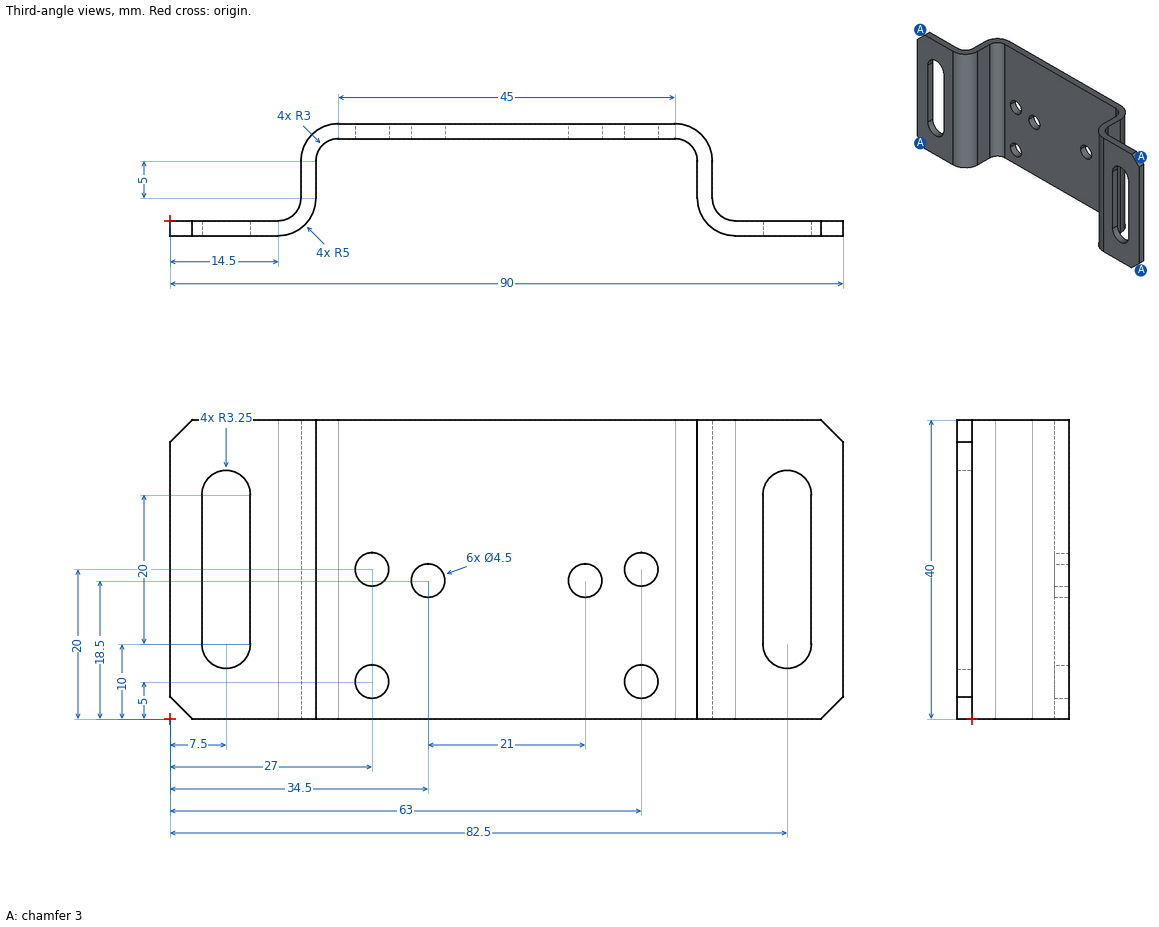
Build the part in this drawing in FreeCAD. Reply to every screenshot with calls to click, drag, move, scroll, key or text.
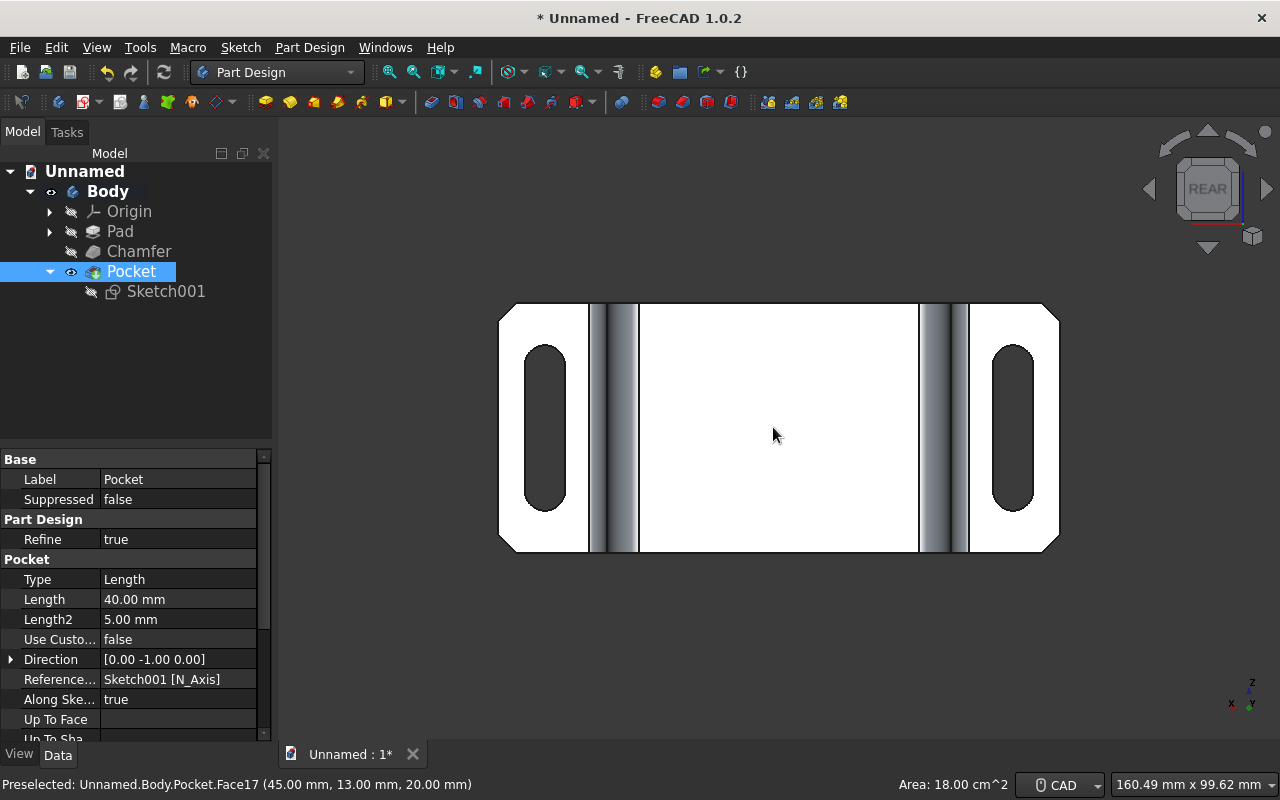
click(84, 102)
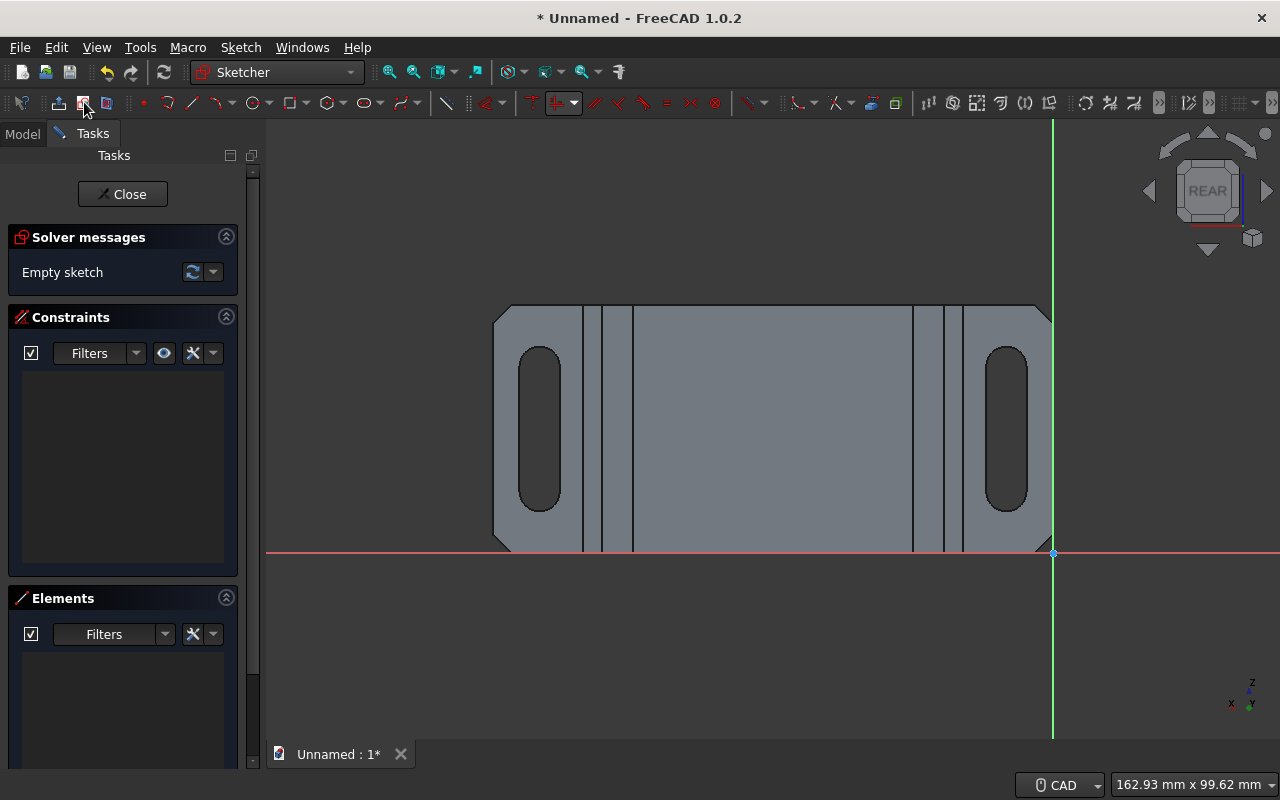
scroll(1115, 597, up, 2)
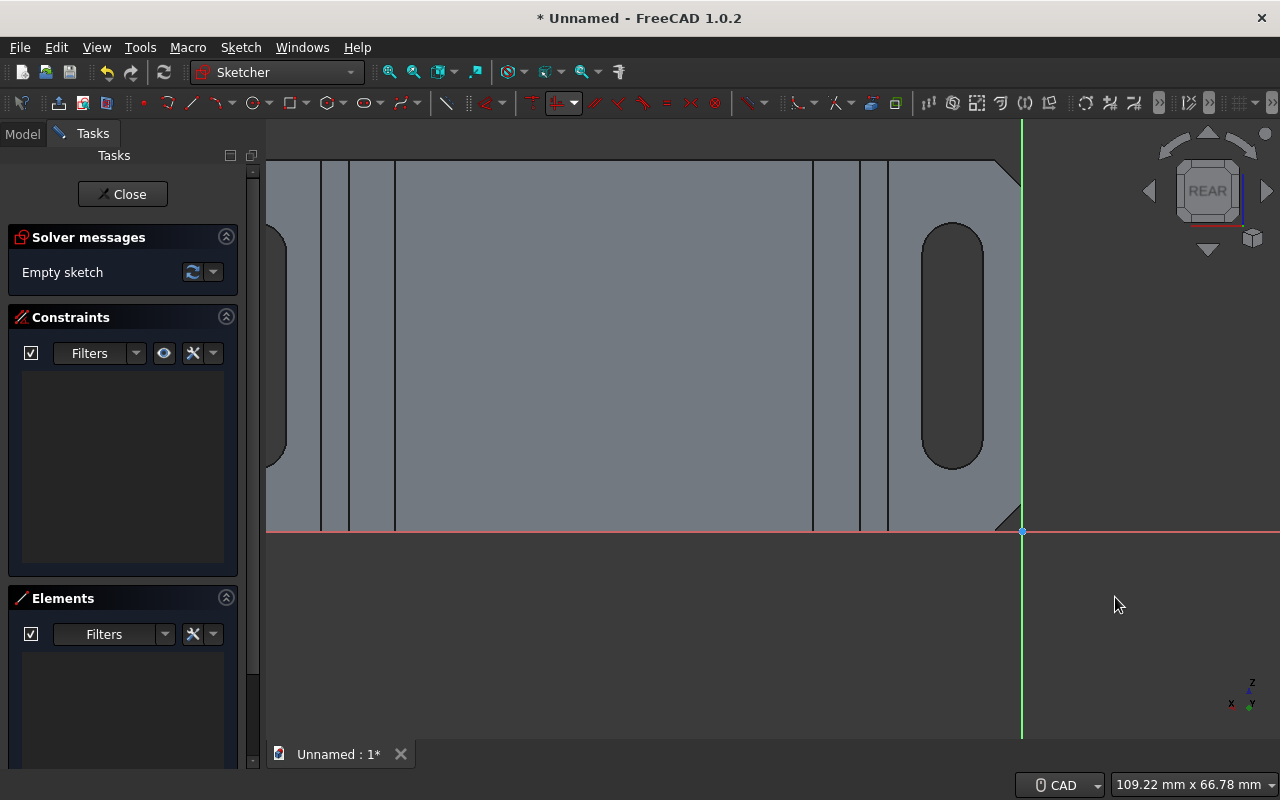
key(g)
key(c)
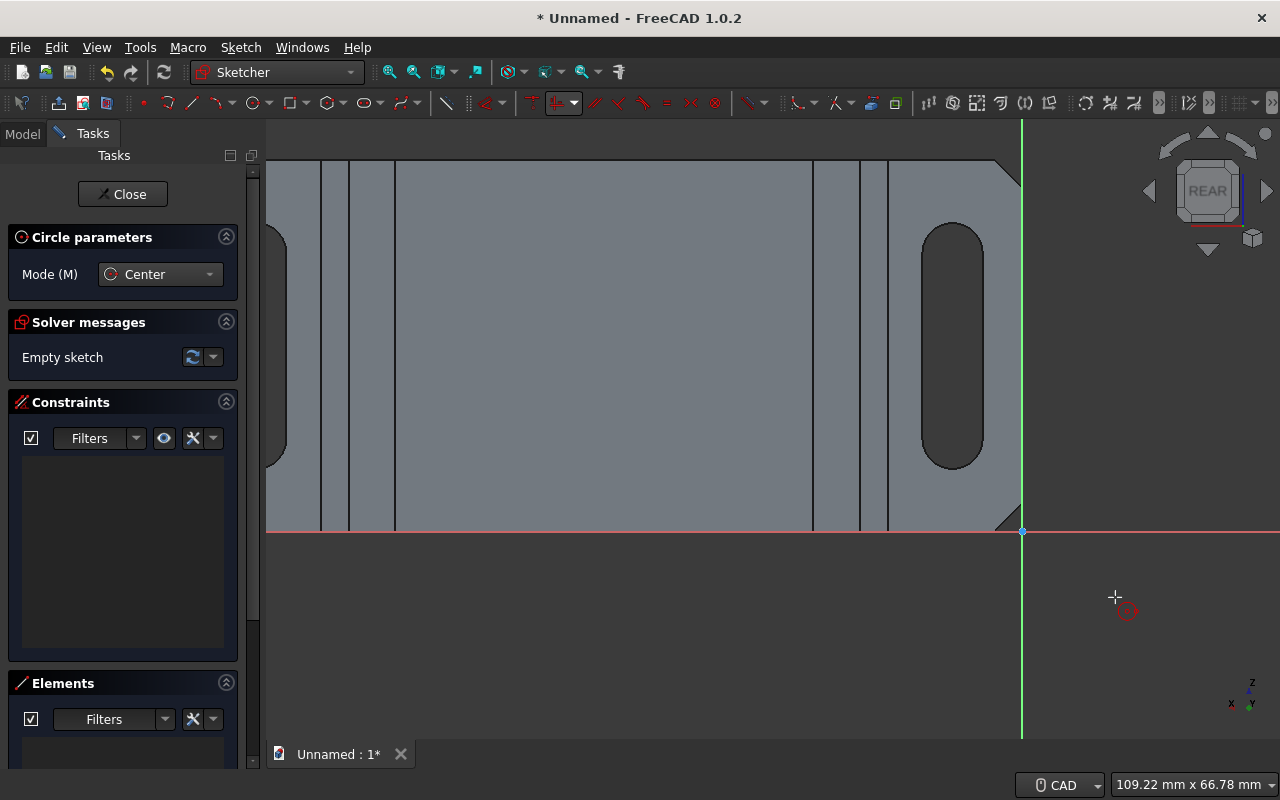
click(702, 360)
move(717, 345)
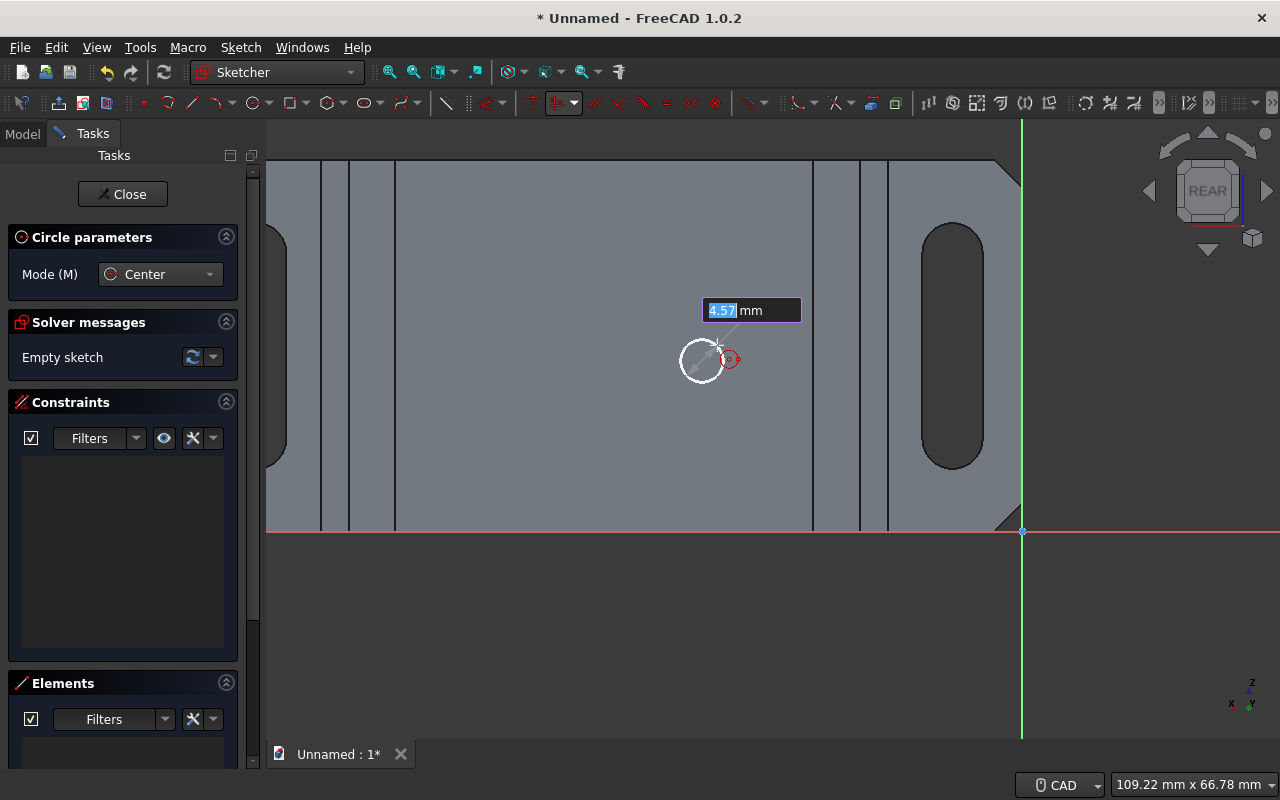
text(4.5)
key(Return)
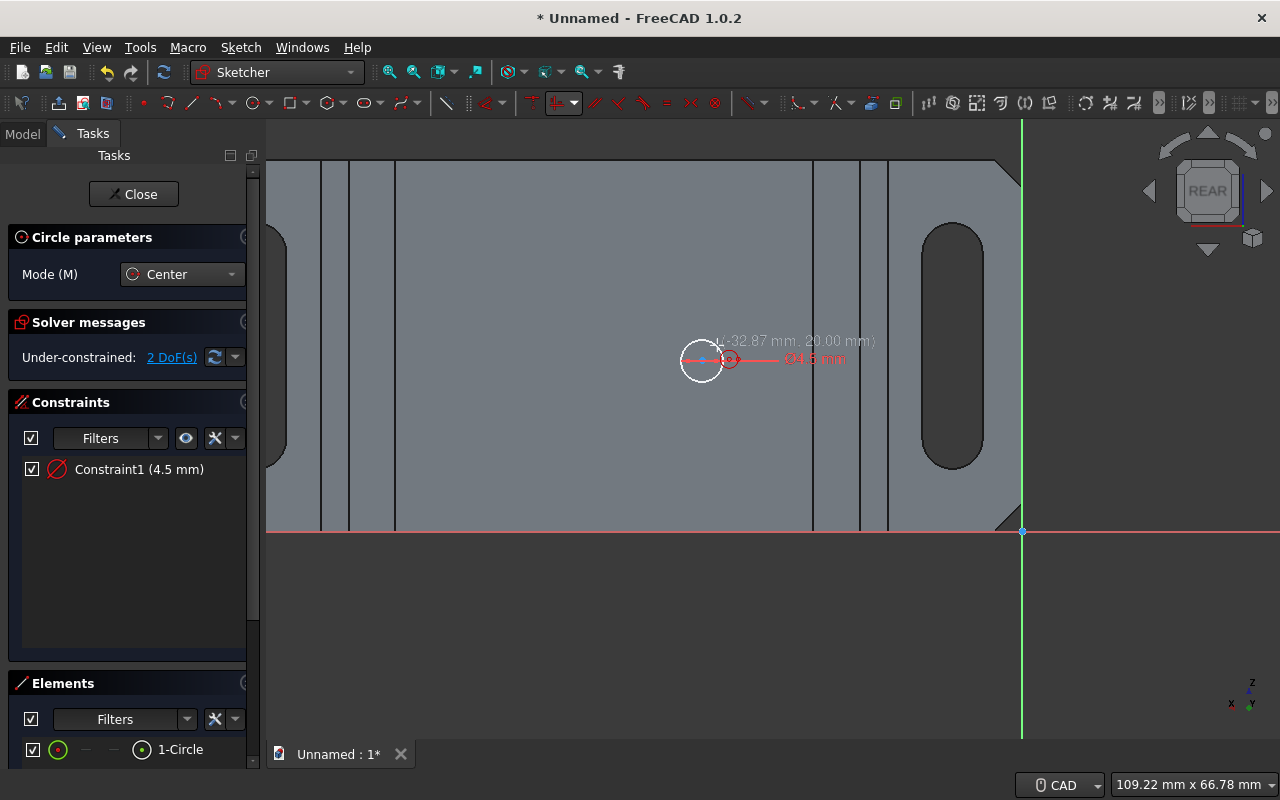
click(771, 346)
move(786, 331)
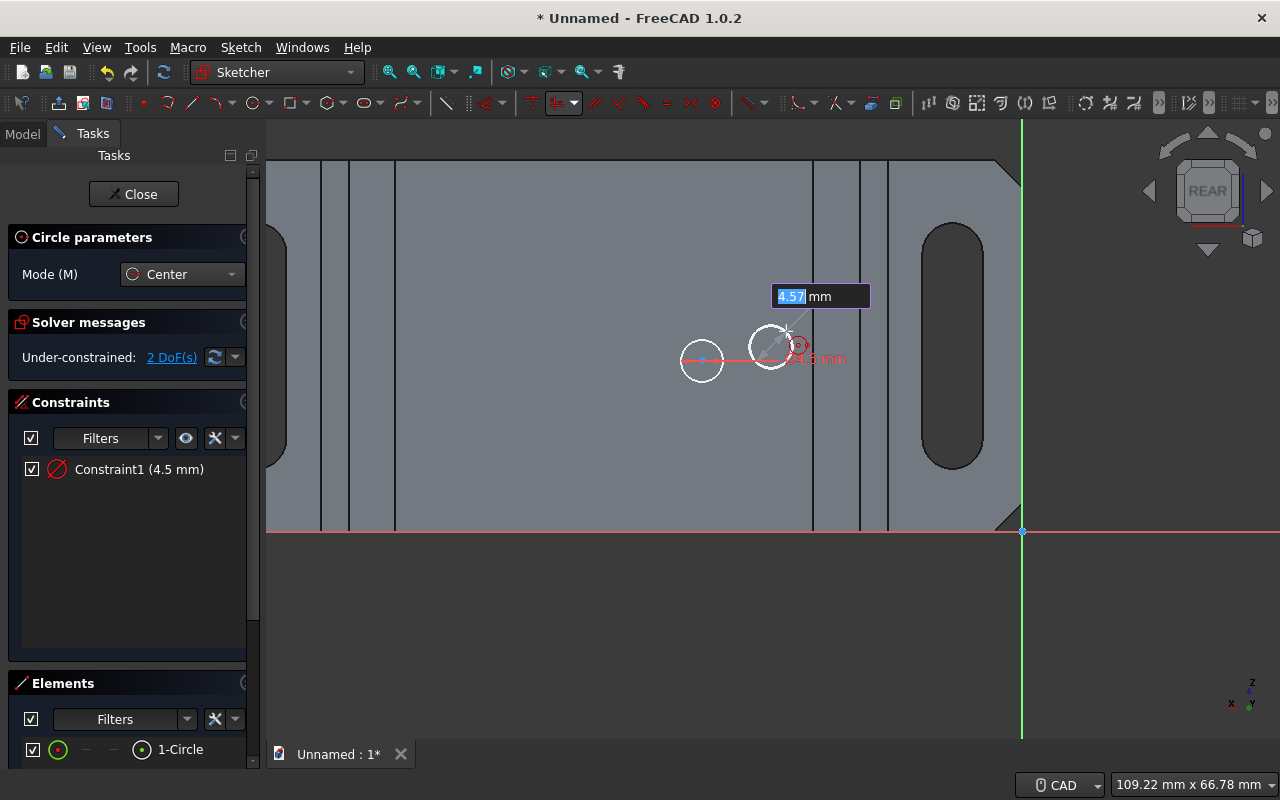
text(4.5)
key(Return)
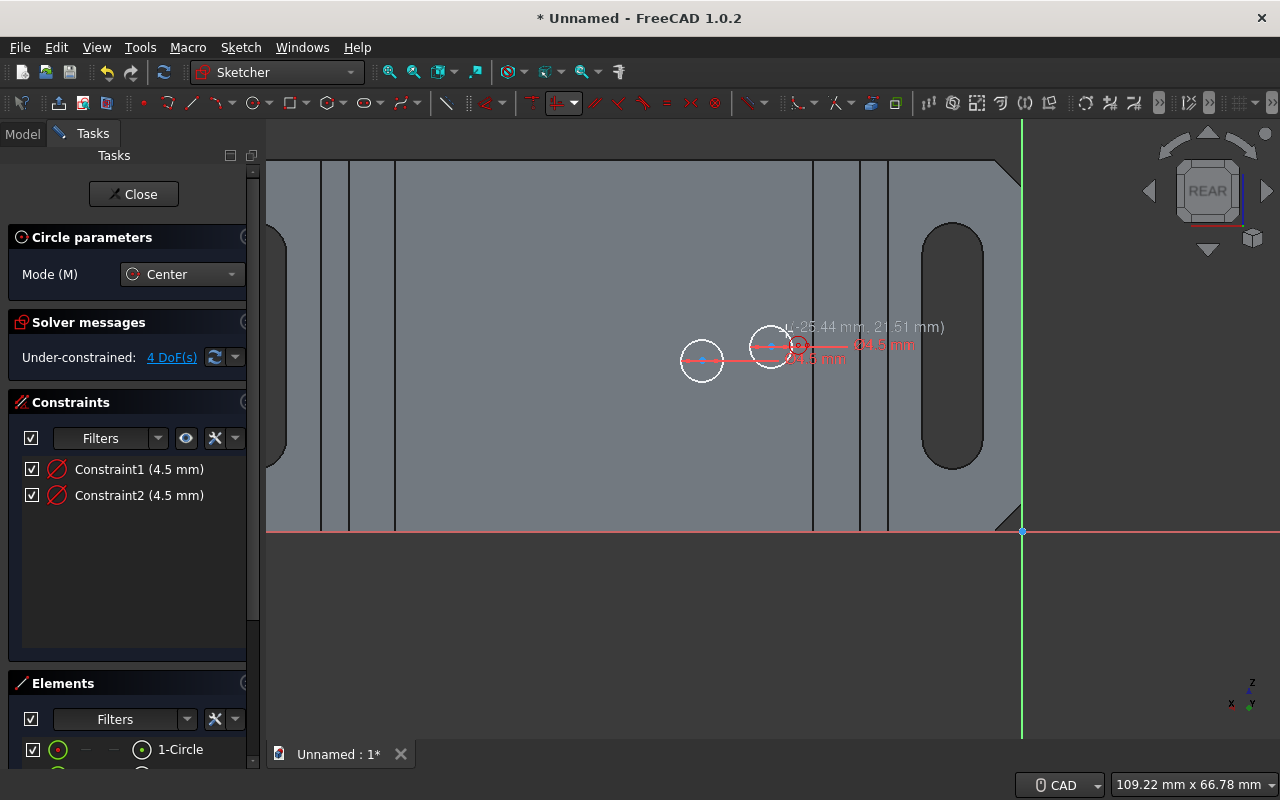
click(507, 360)
move(522, 345)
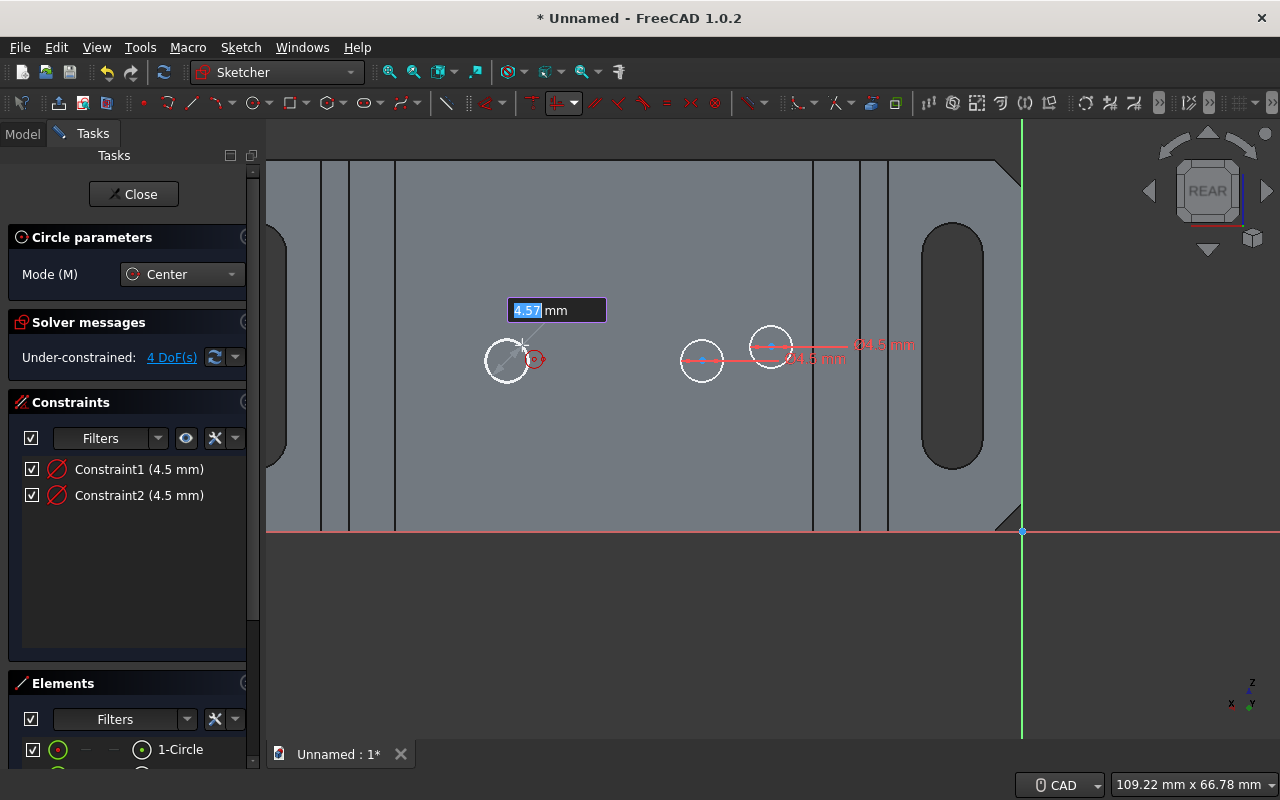
text(4.5)
key(Return)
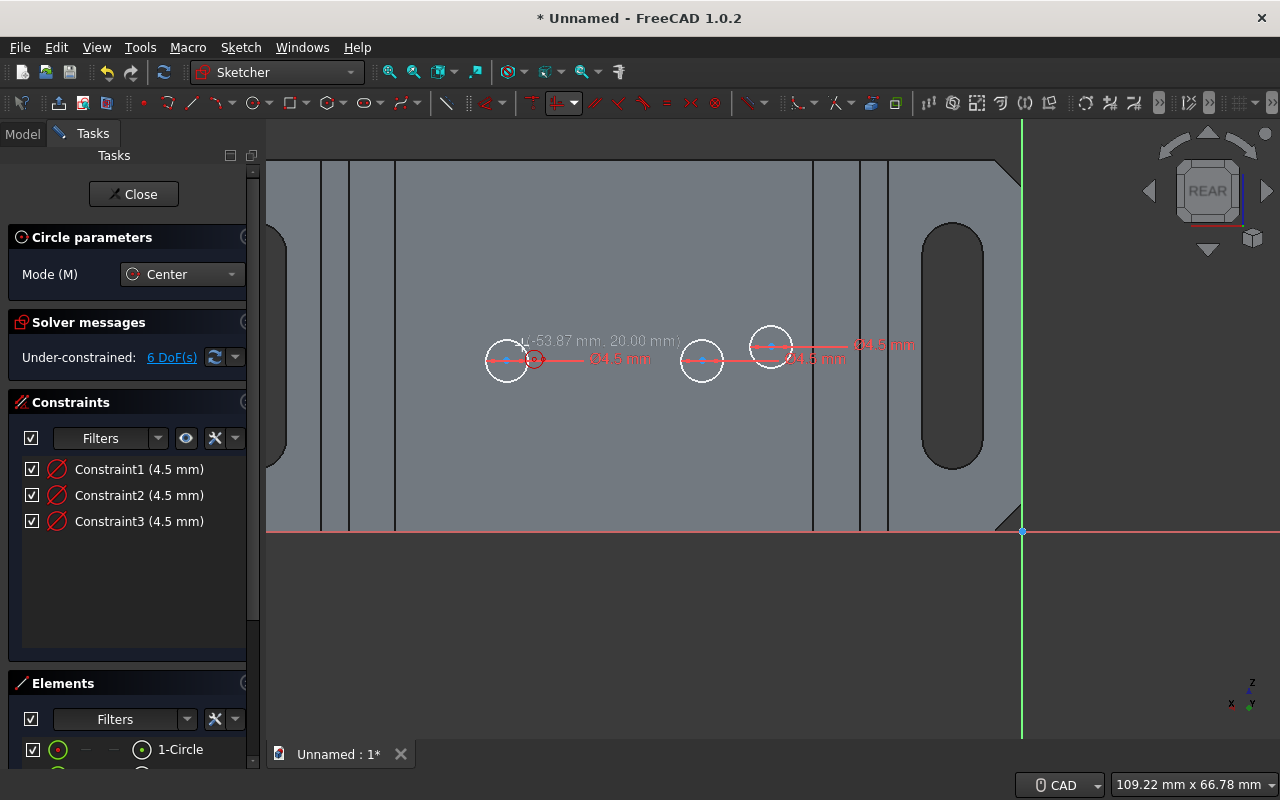
click(437, 346)
move(452, 331)